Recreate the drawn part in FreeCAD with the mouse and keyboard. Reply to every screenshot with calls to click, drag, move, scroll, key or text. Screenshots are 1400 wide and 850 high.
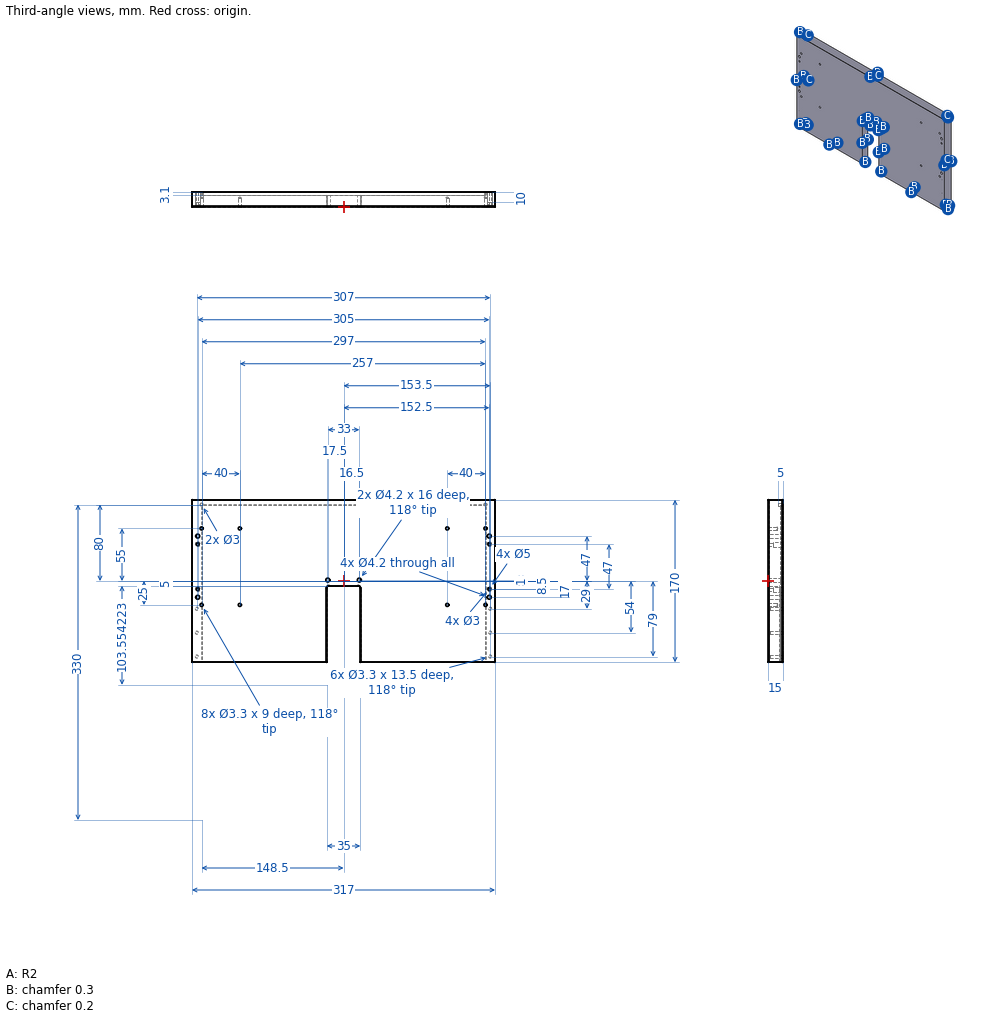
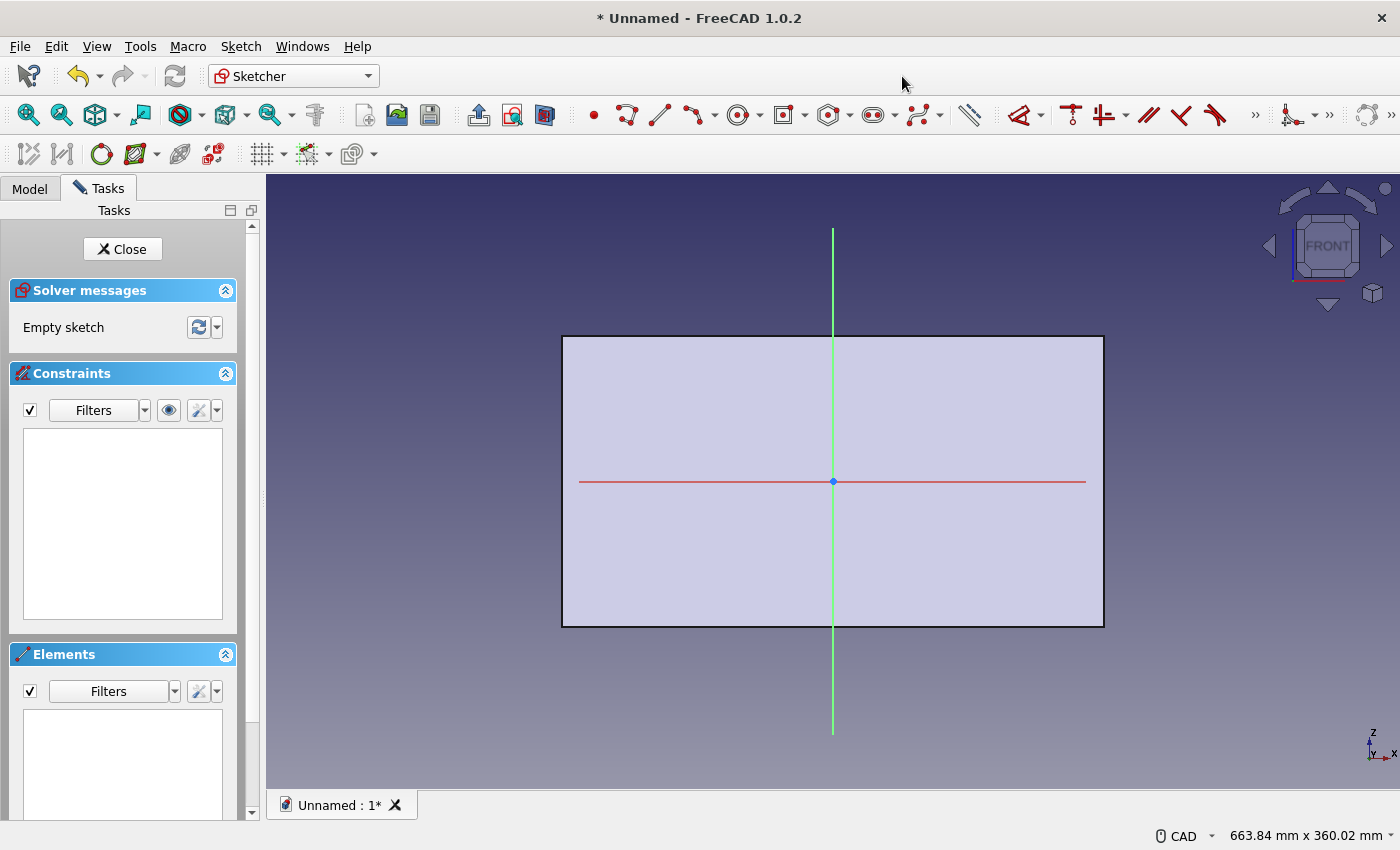
scroll(889, 650, up, 4)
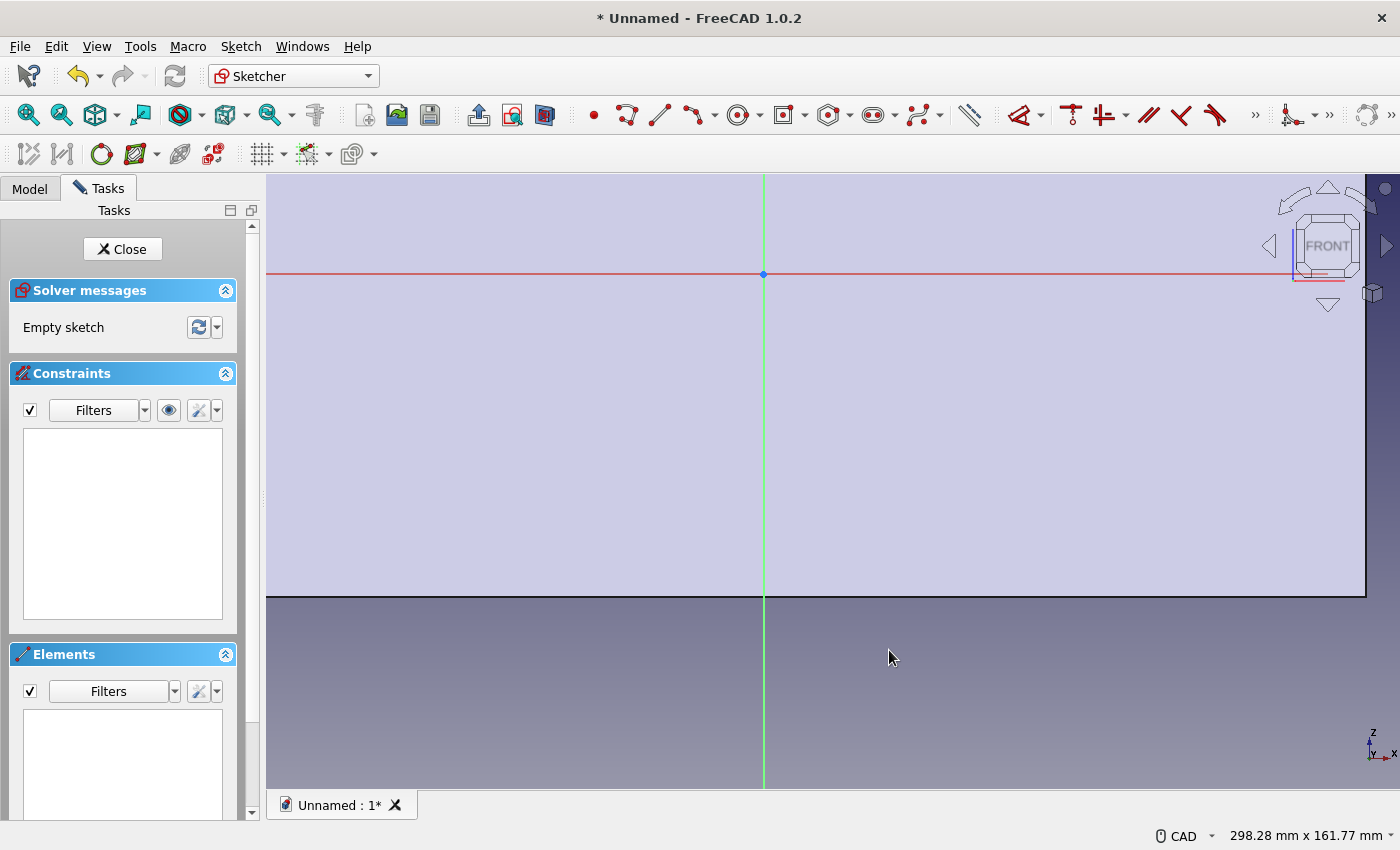
key(g)
key(r)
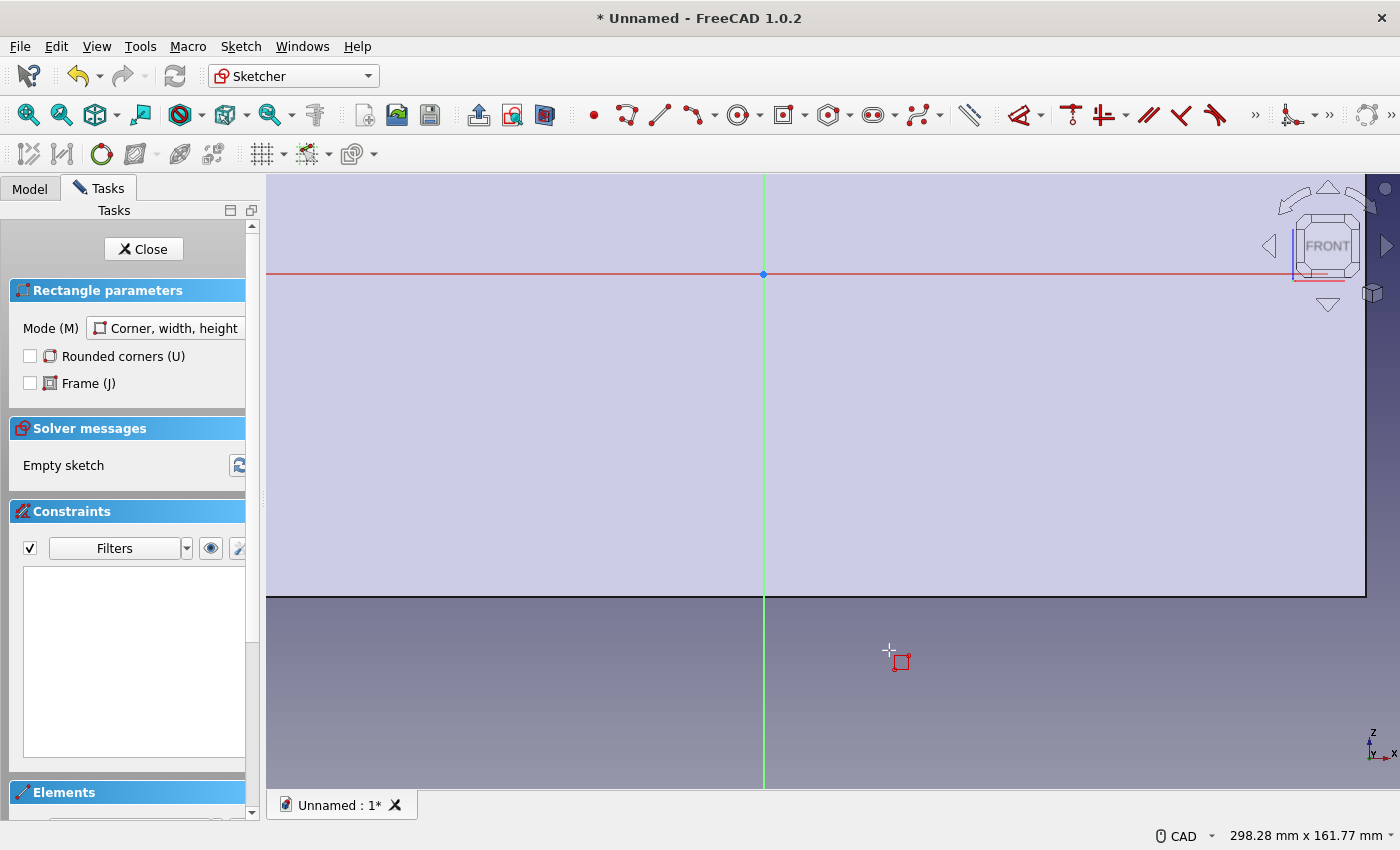
click(697, 293)
click(830, 687)
key(Escape)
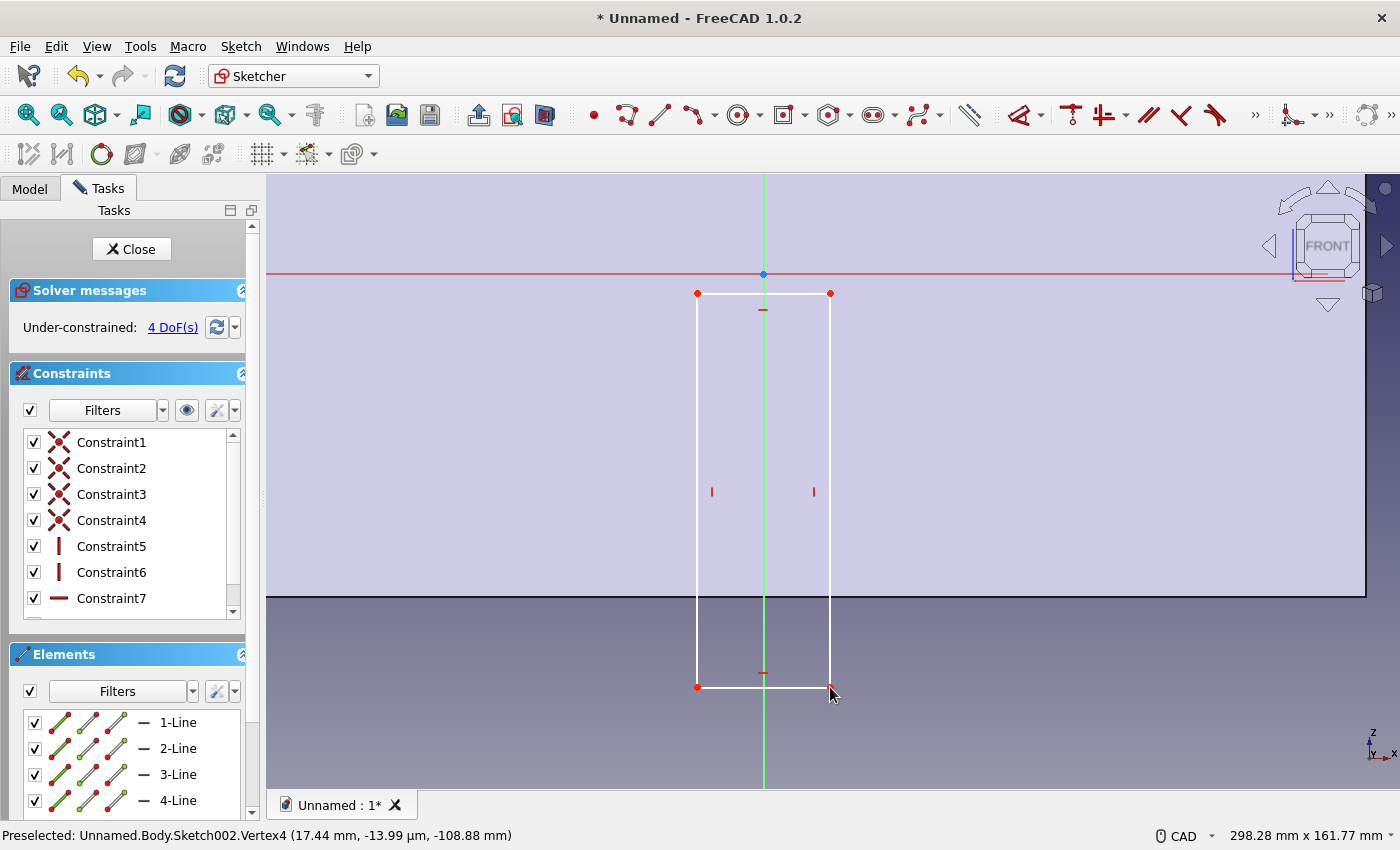
key(d)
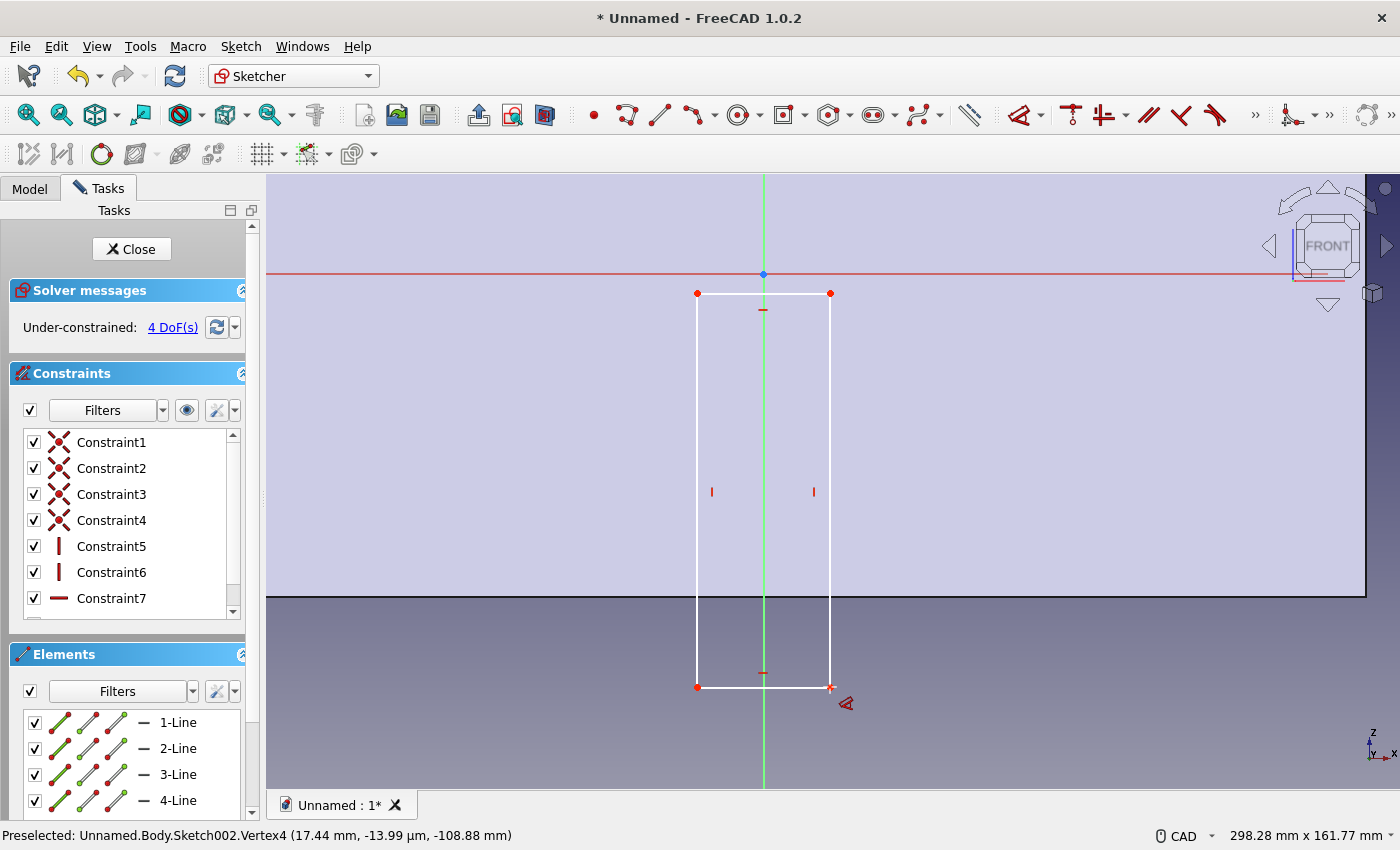
click(737, 688)
click(733, 722)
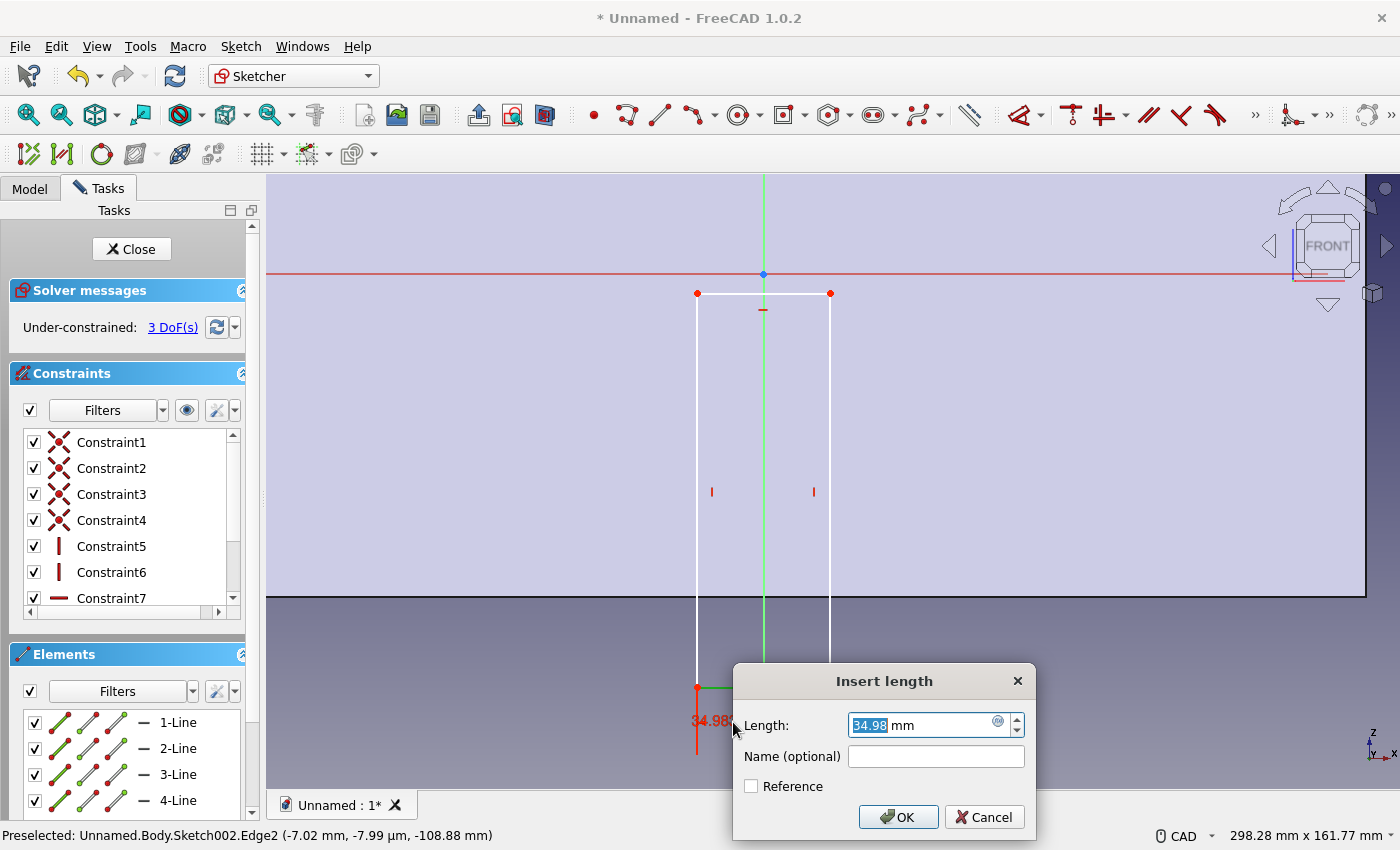
text(35)
key(Return)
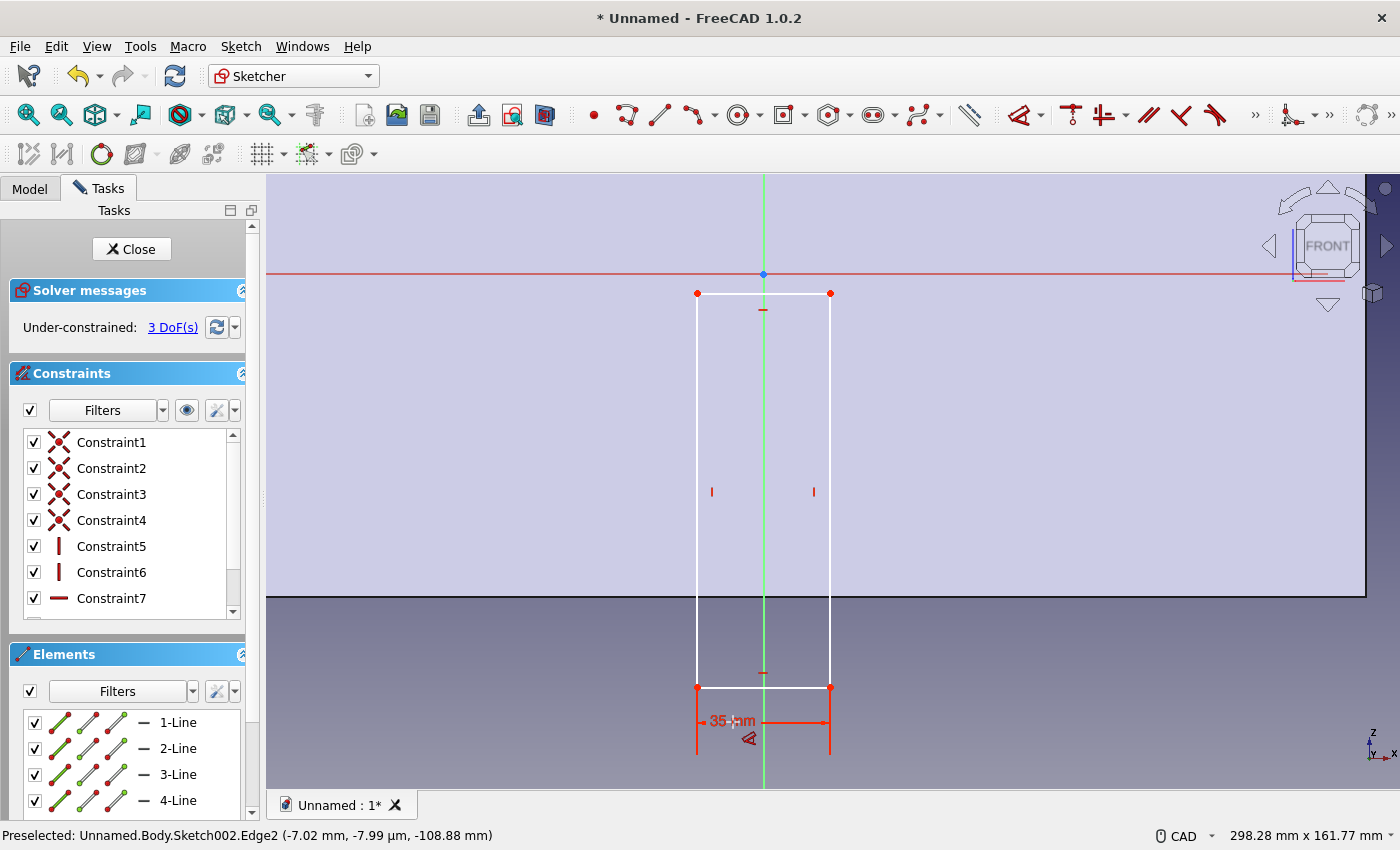
scroll(697, 294, up, 4)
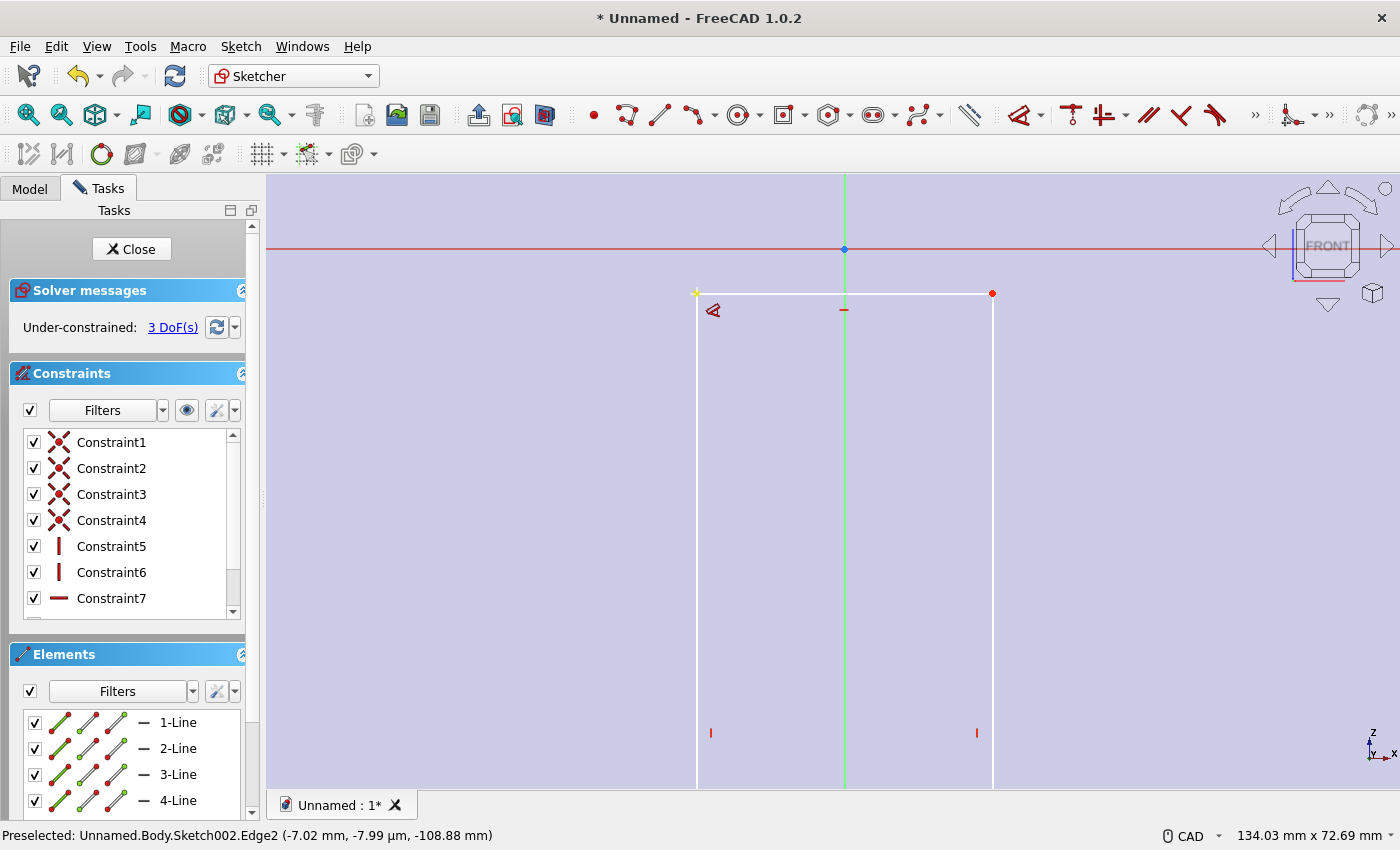
click(697, 294)
click(663, 272)